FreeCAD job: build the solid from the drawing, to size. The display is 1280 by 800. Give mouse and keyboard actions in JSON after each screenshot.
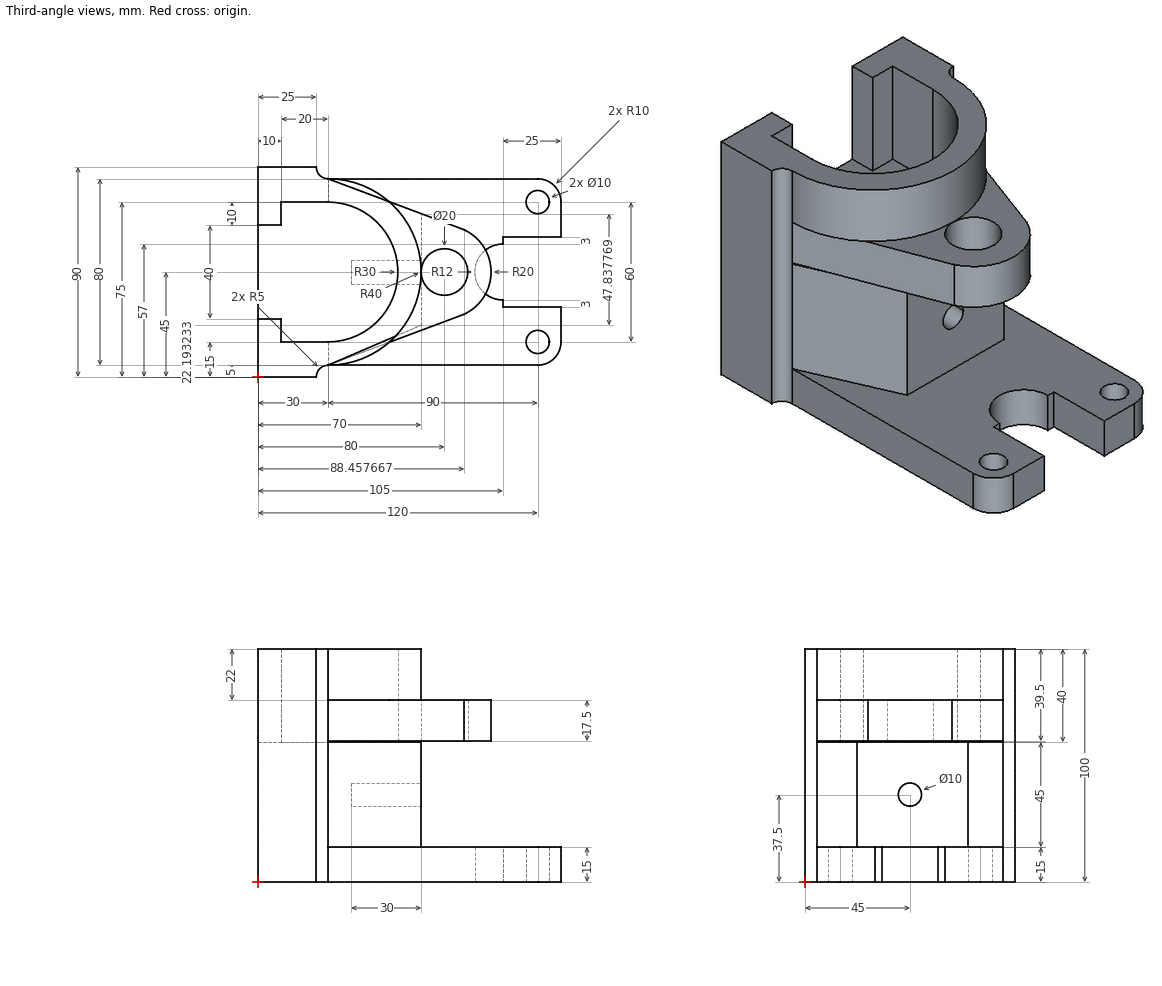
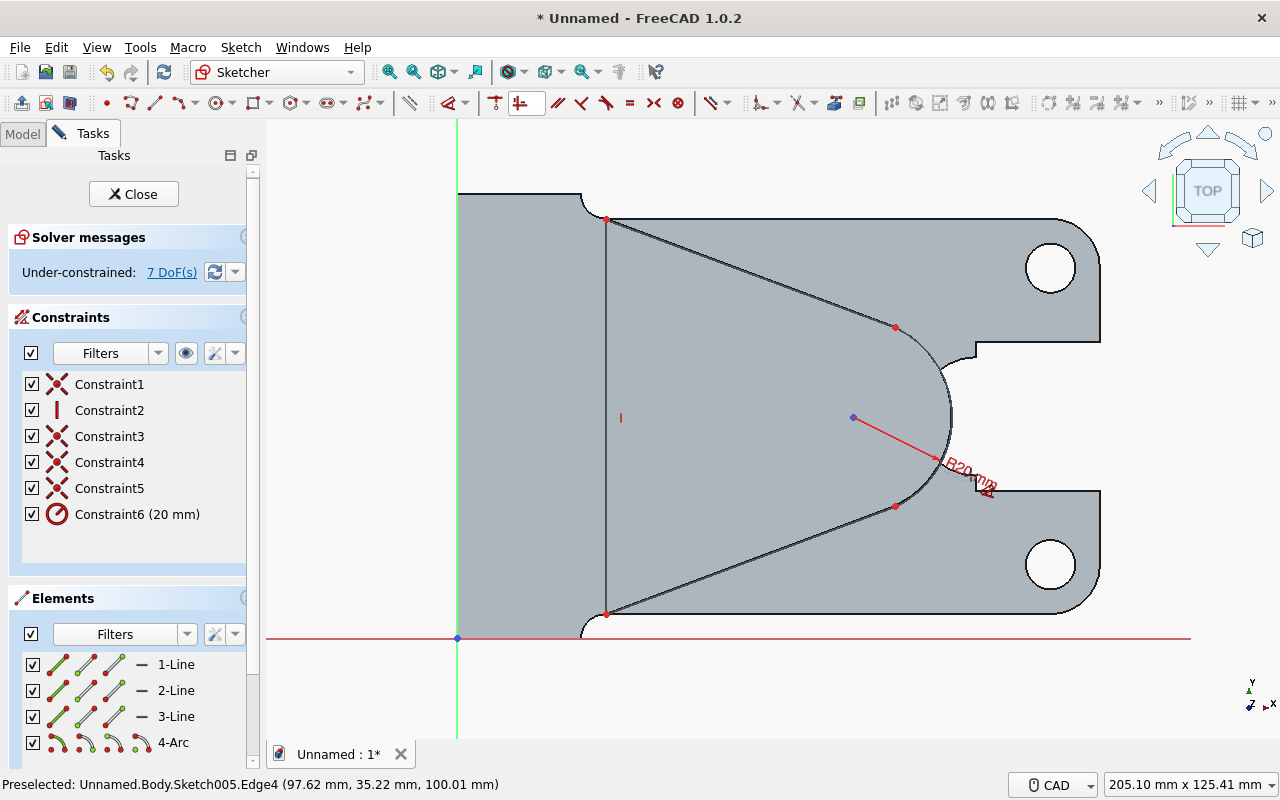
{"action": "left_click", "coordinate": [606, 339]}
{"action": "left_click", "coordinate": [572, 418]}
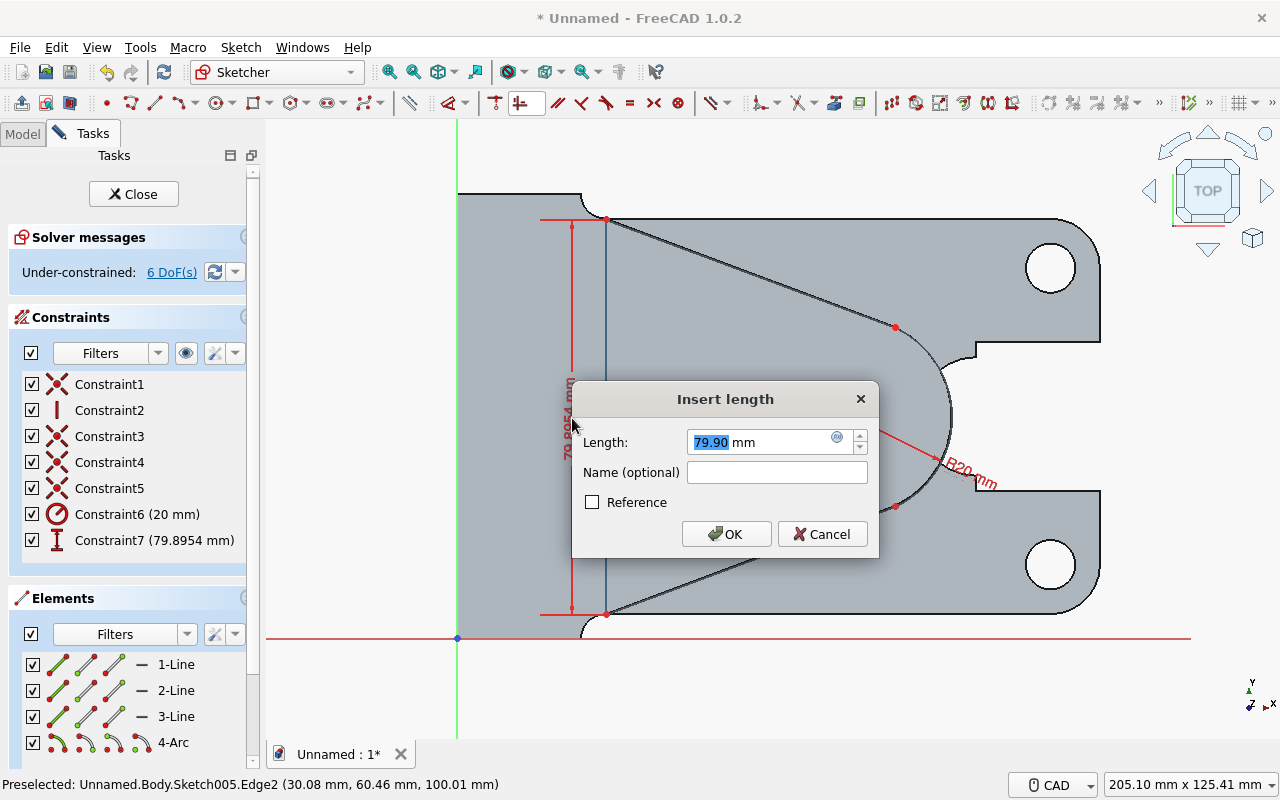
{"action": "type", "text": "80"}
{"action": "key", "text": "Return"}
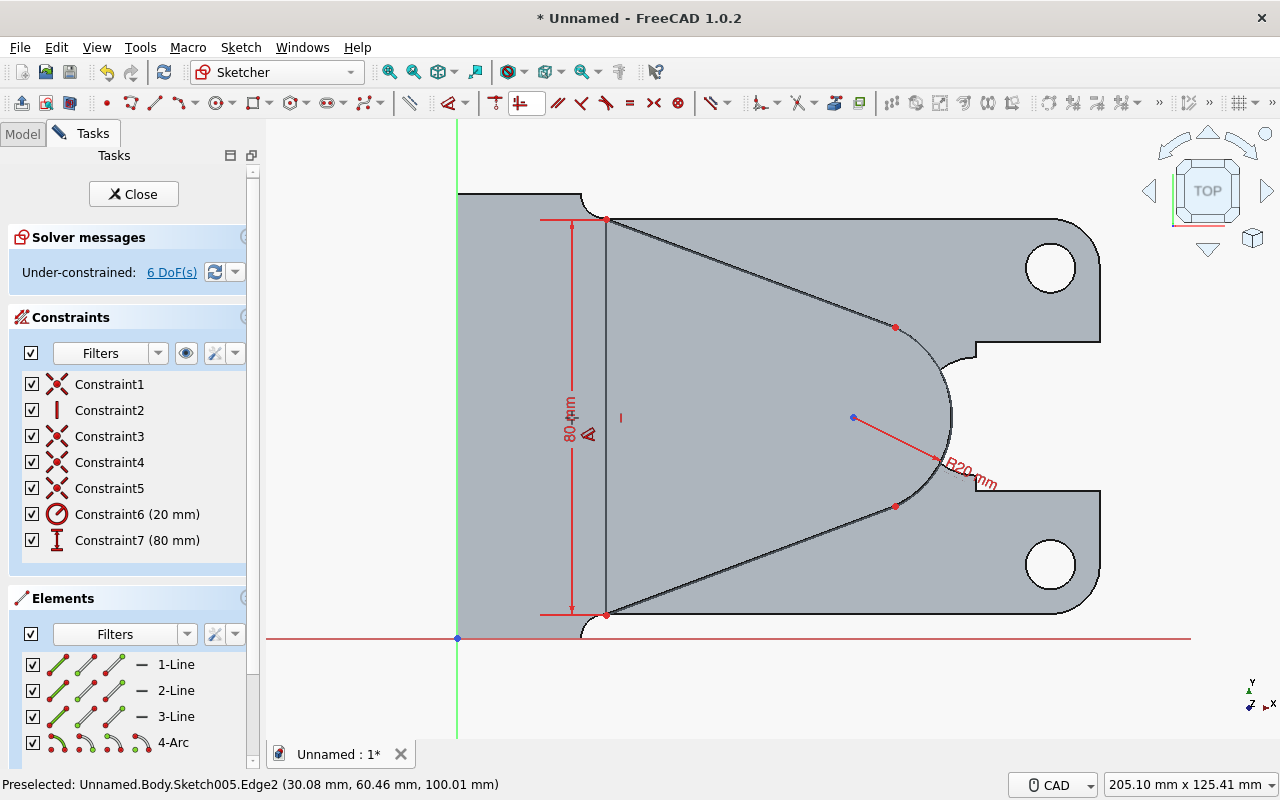
{"action": "scroll", "coordinate": [606, 615], "scroll_direction": "up", "scroll_amount": 3}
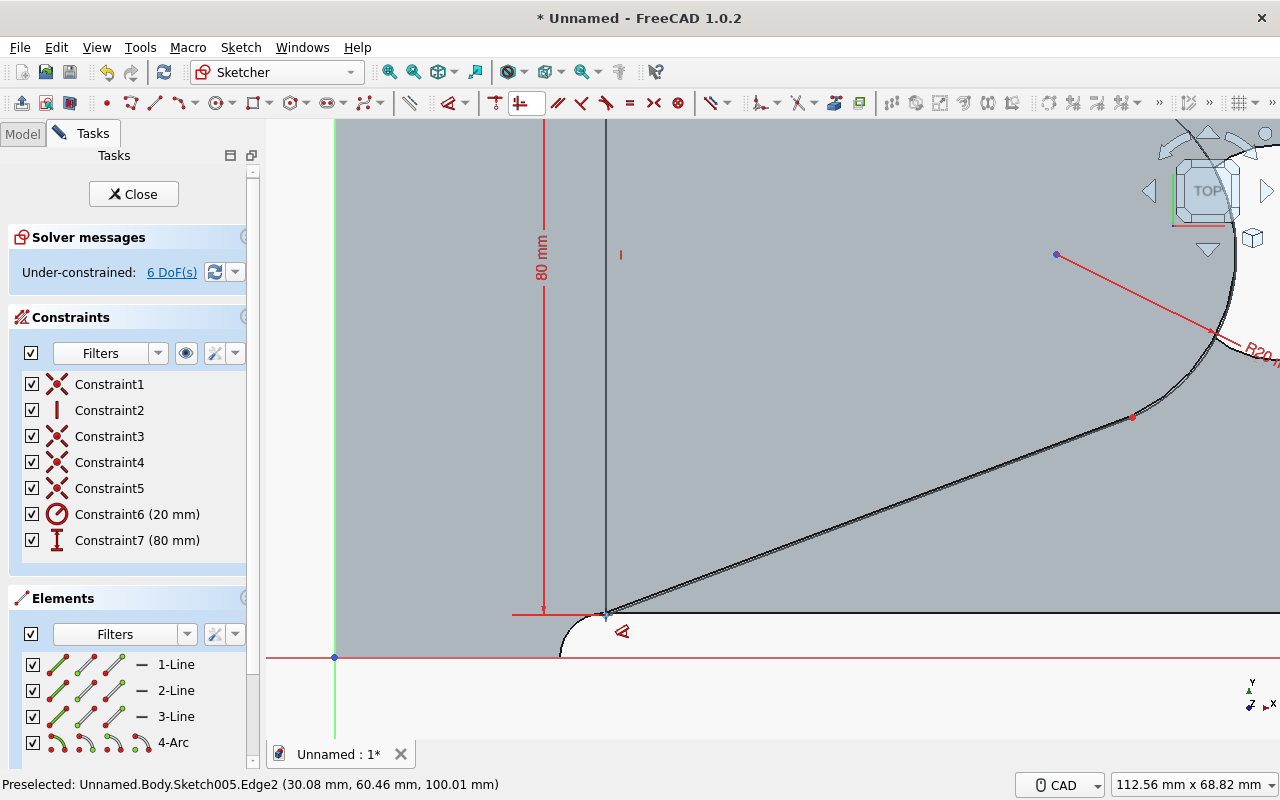
{"action": "left_click", "coordinate": [606, 615]}
{"action": "left_click", "coordinate": [301, 637]}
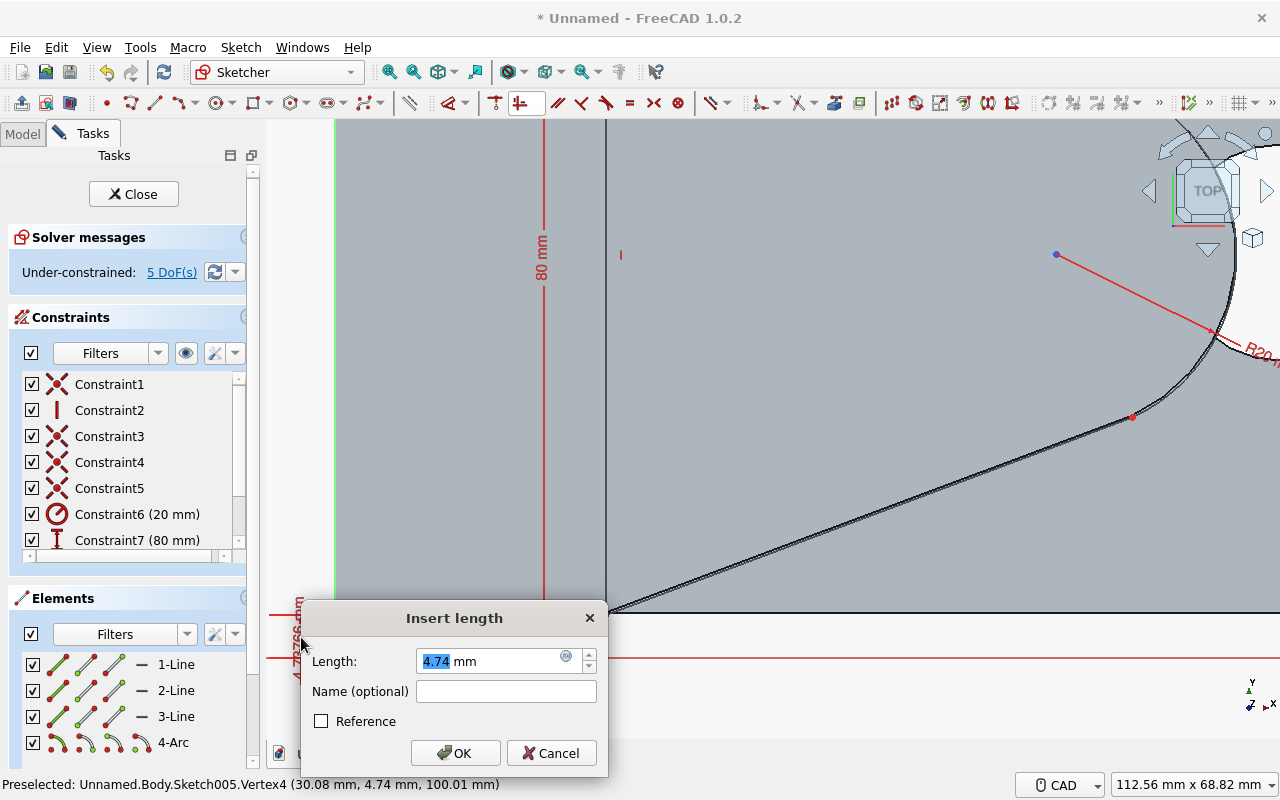
{"action": "type", "text": "5"}
{"action": "key", "text": "Return"}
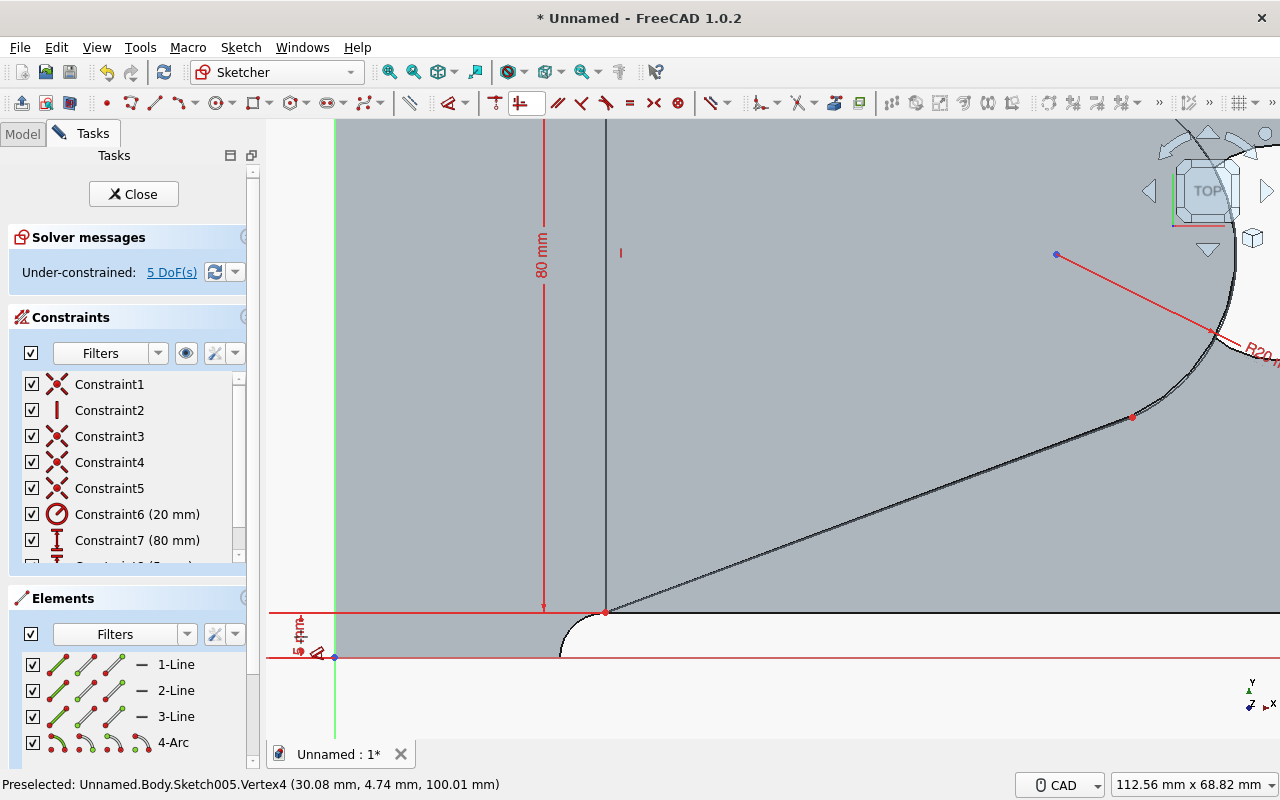
{"action": "scroll", "coordinate": [606, 616], "scroll_direction": "down", "scroll_amount": 3}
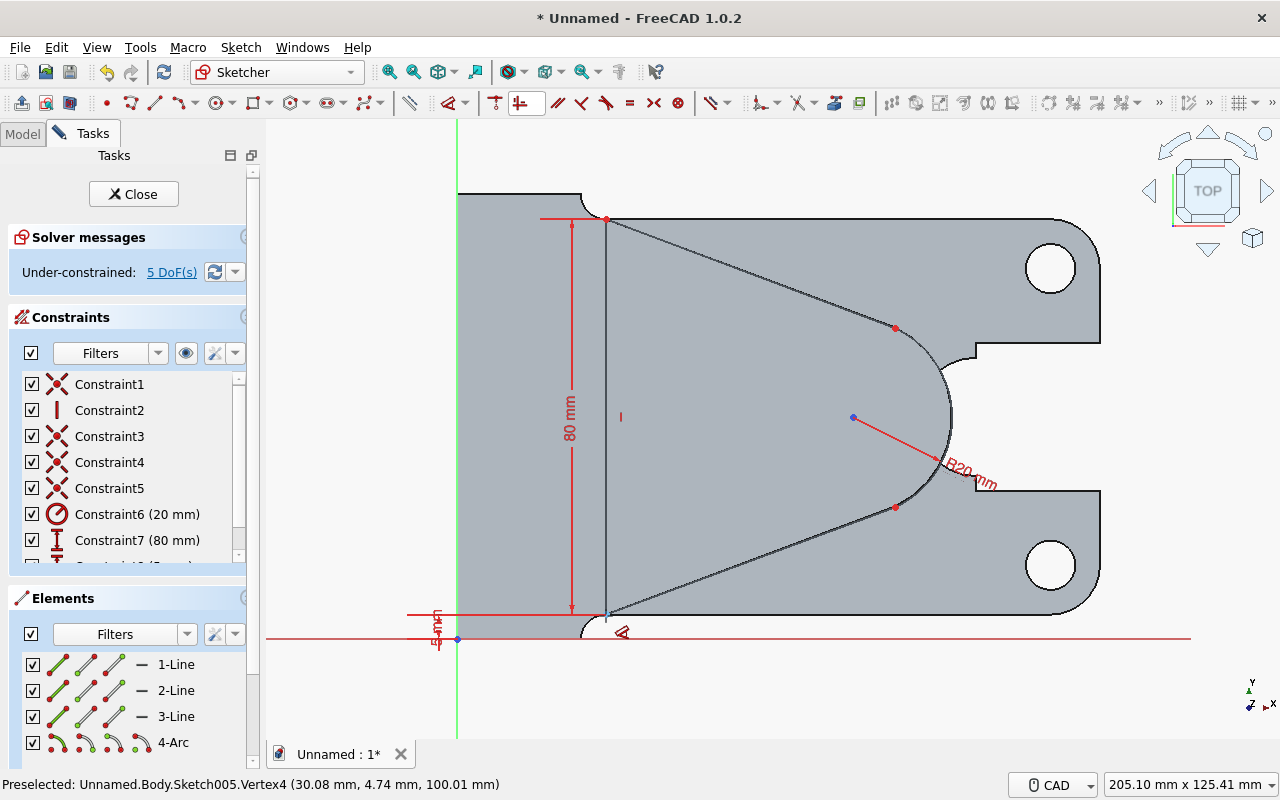
{"action": "left_click", "coordinate": [606, 219]}
{"action": "left_click", "coordinate": [532, 673]}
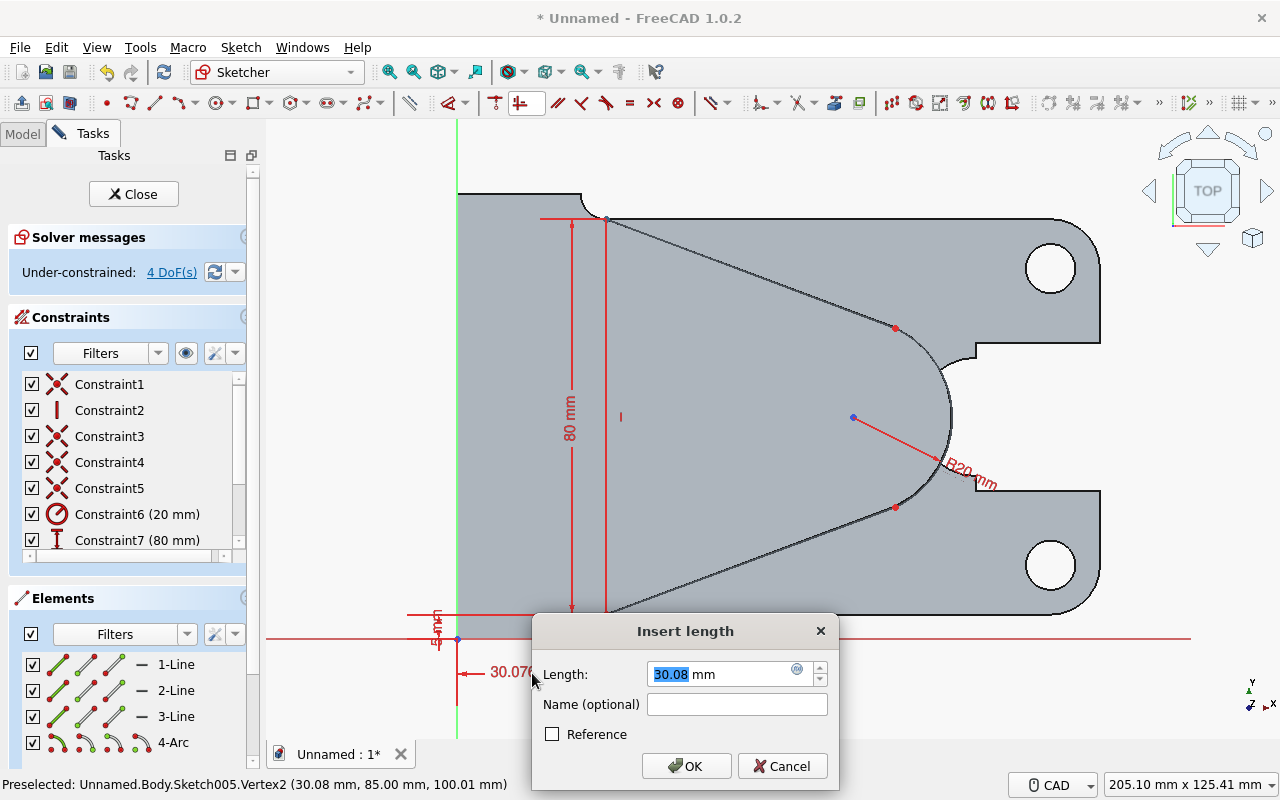
{"action": "type", "text": "30"}
{"action": "key", "text": "Return"}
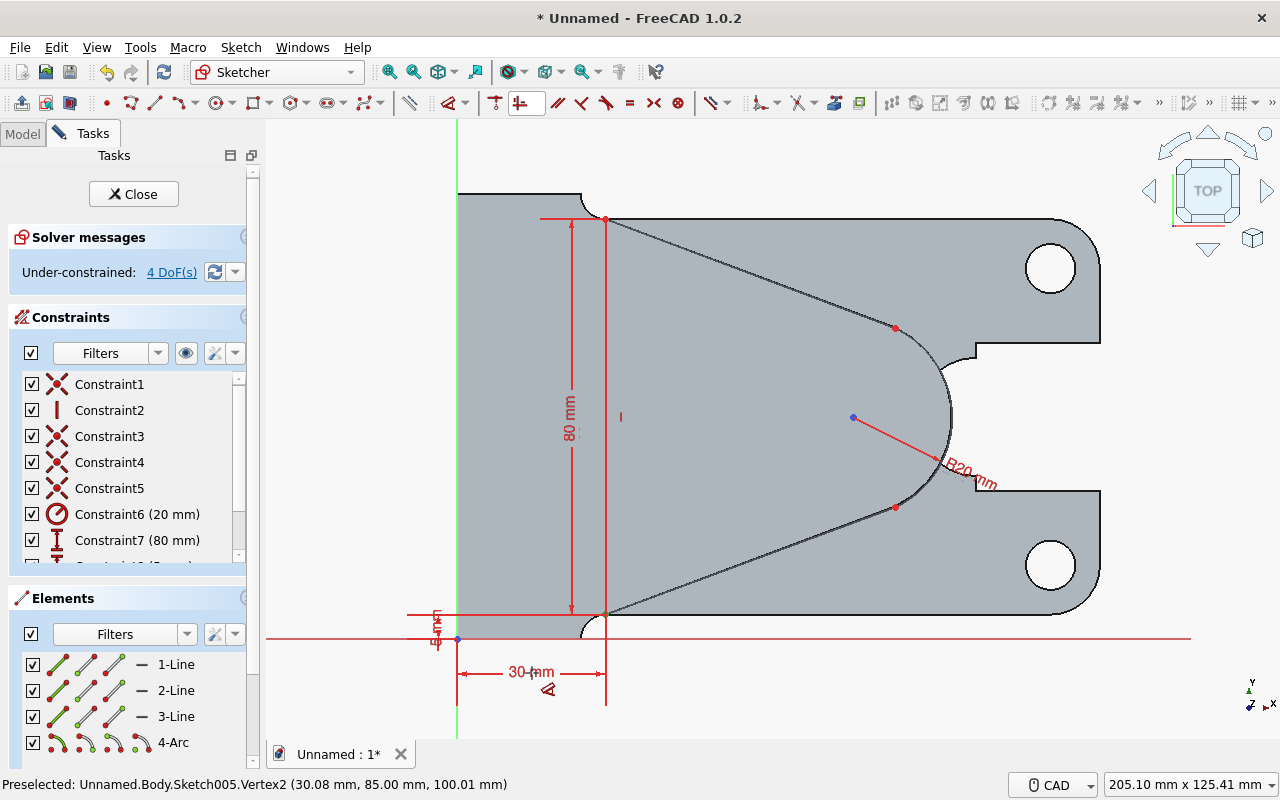
{"action": "left_click", "coordinate": [853, 418]}
{"action": "left_click", "coordinate": [655, 673]}